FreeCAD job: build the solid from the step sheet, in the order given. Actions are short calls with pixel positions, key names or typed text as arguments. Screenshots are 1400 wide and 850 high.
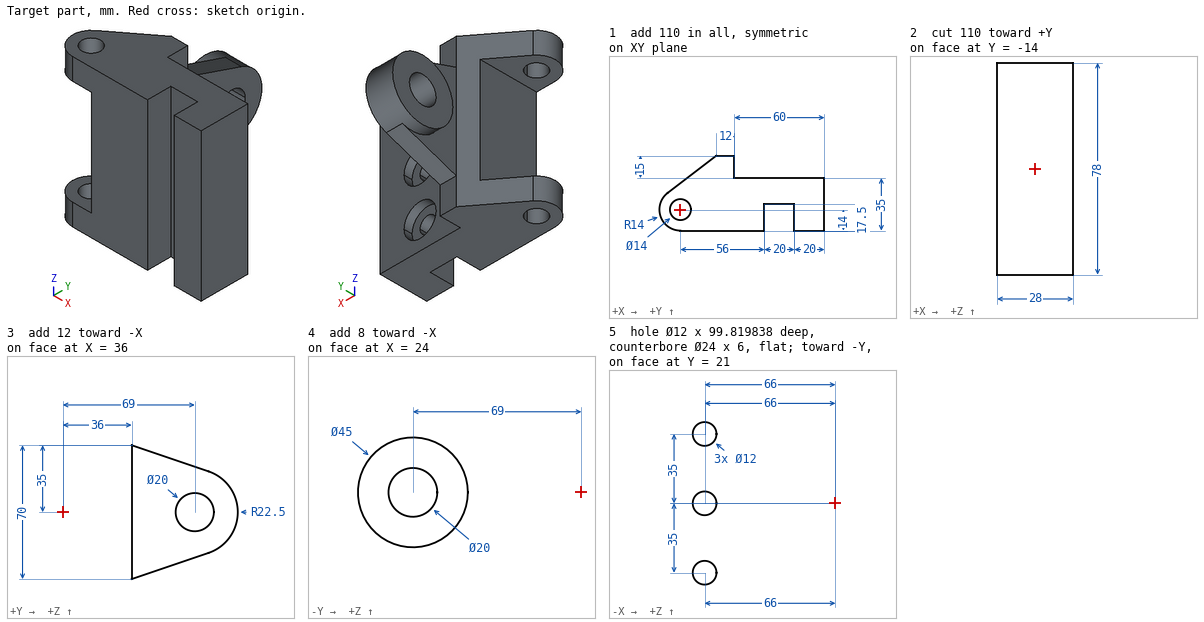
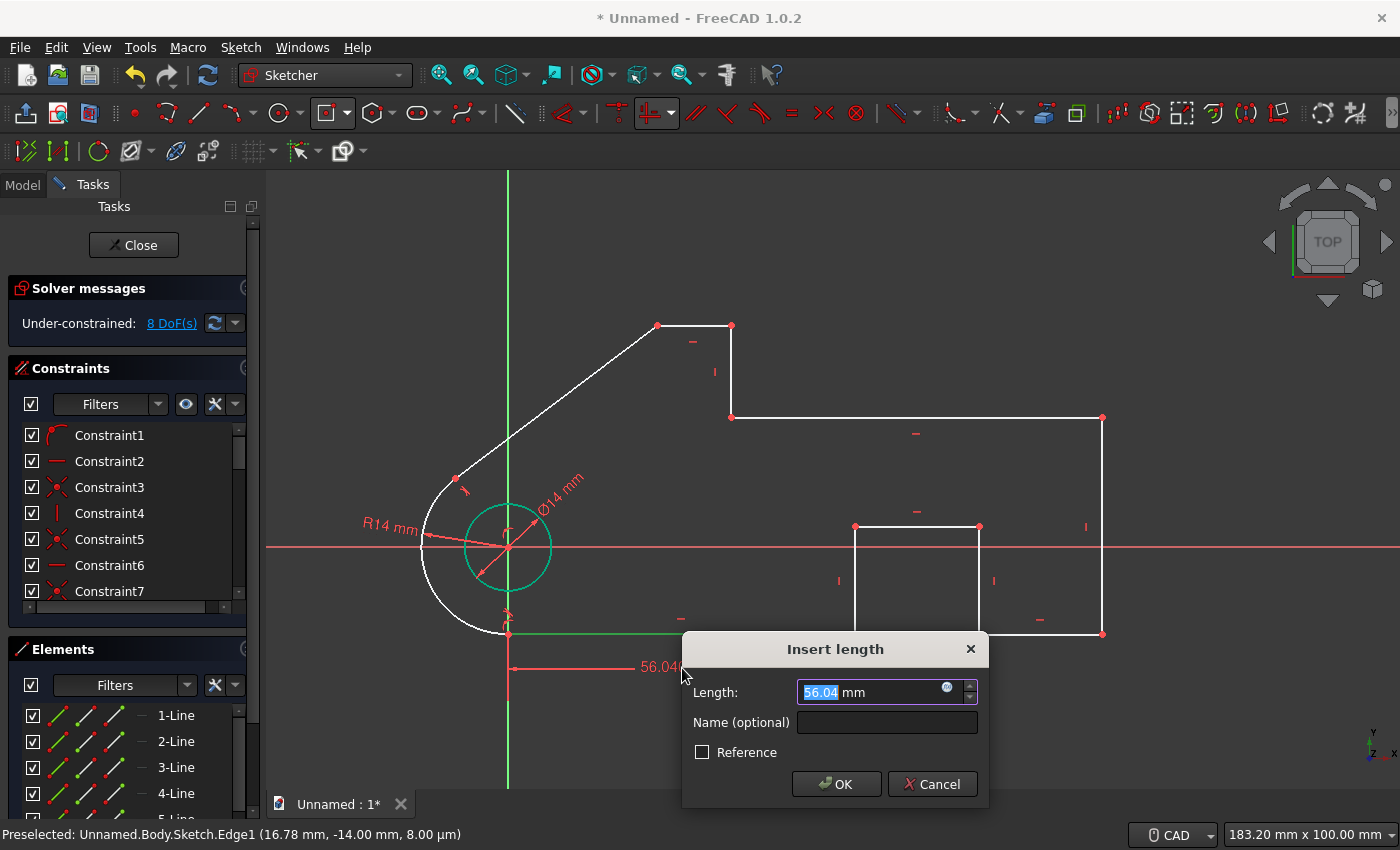
text(56)
key(Return)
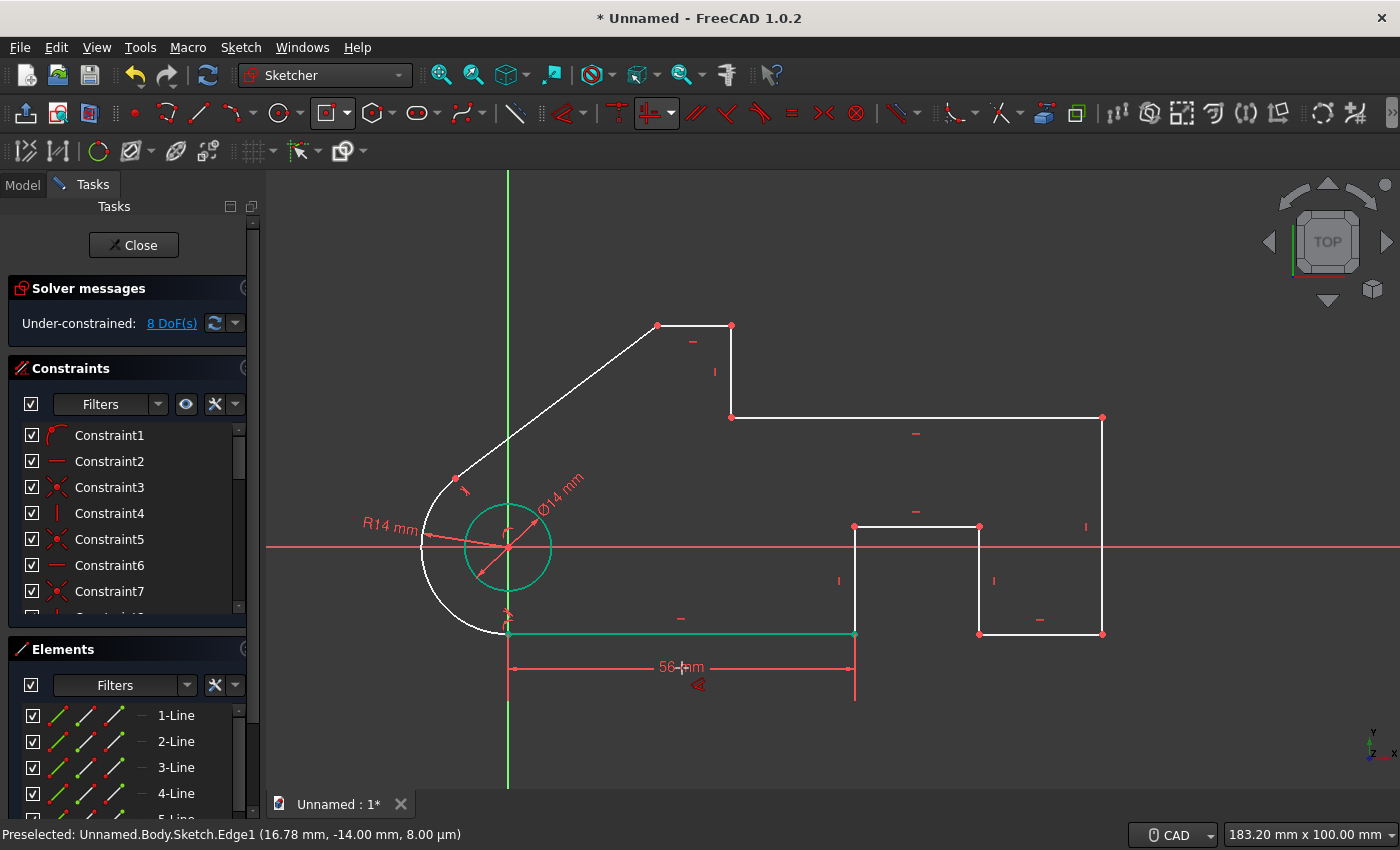
click(892, 527)
click(917, 561)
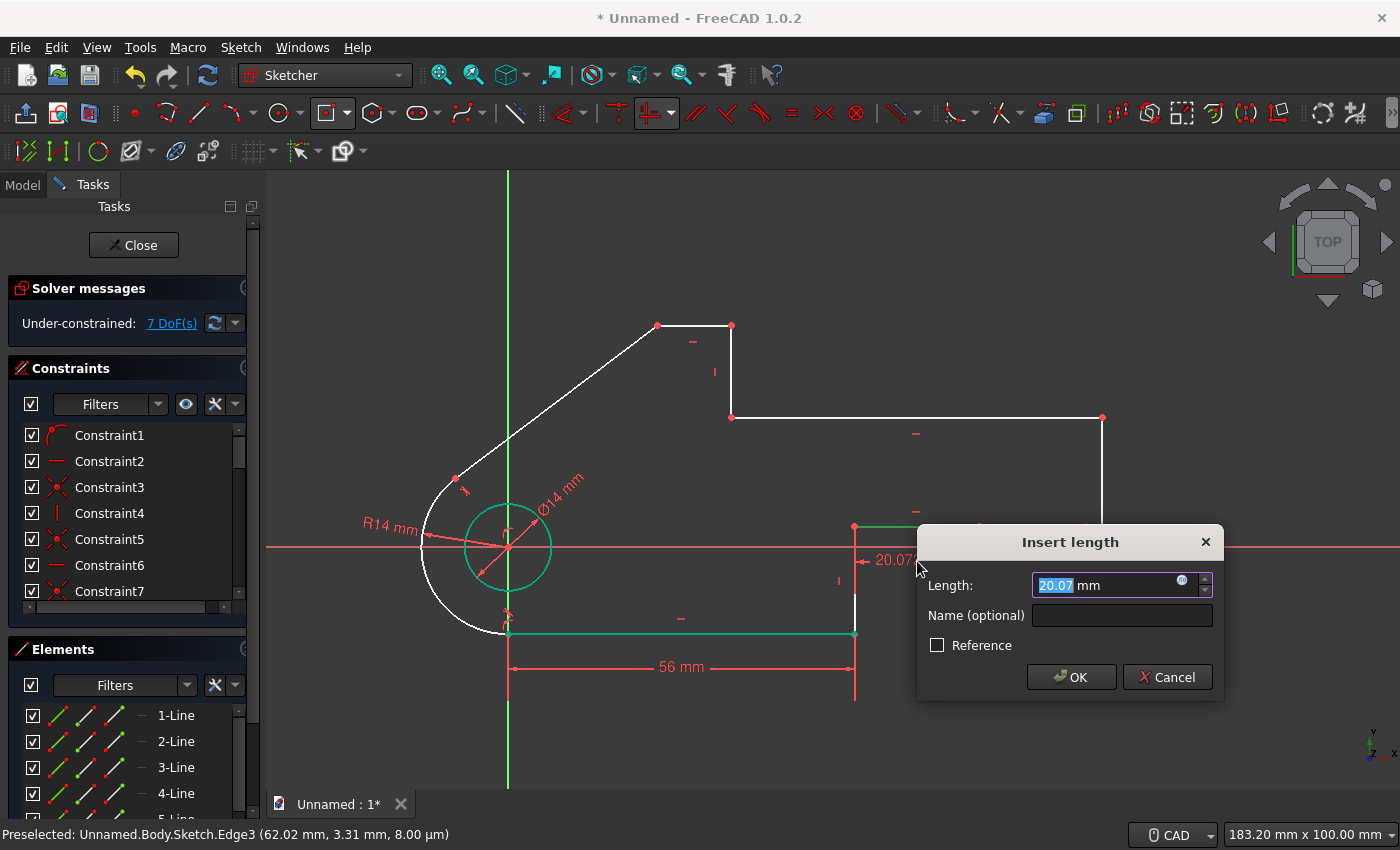
text(20)
key(Return)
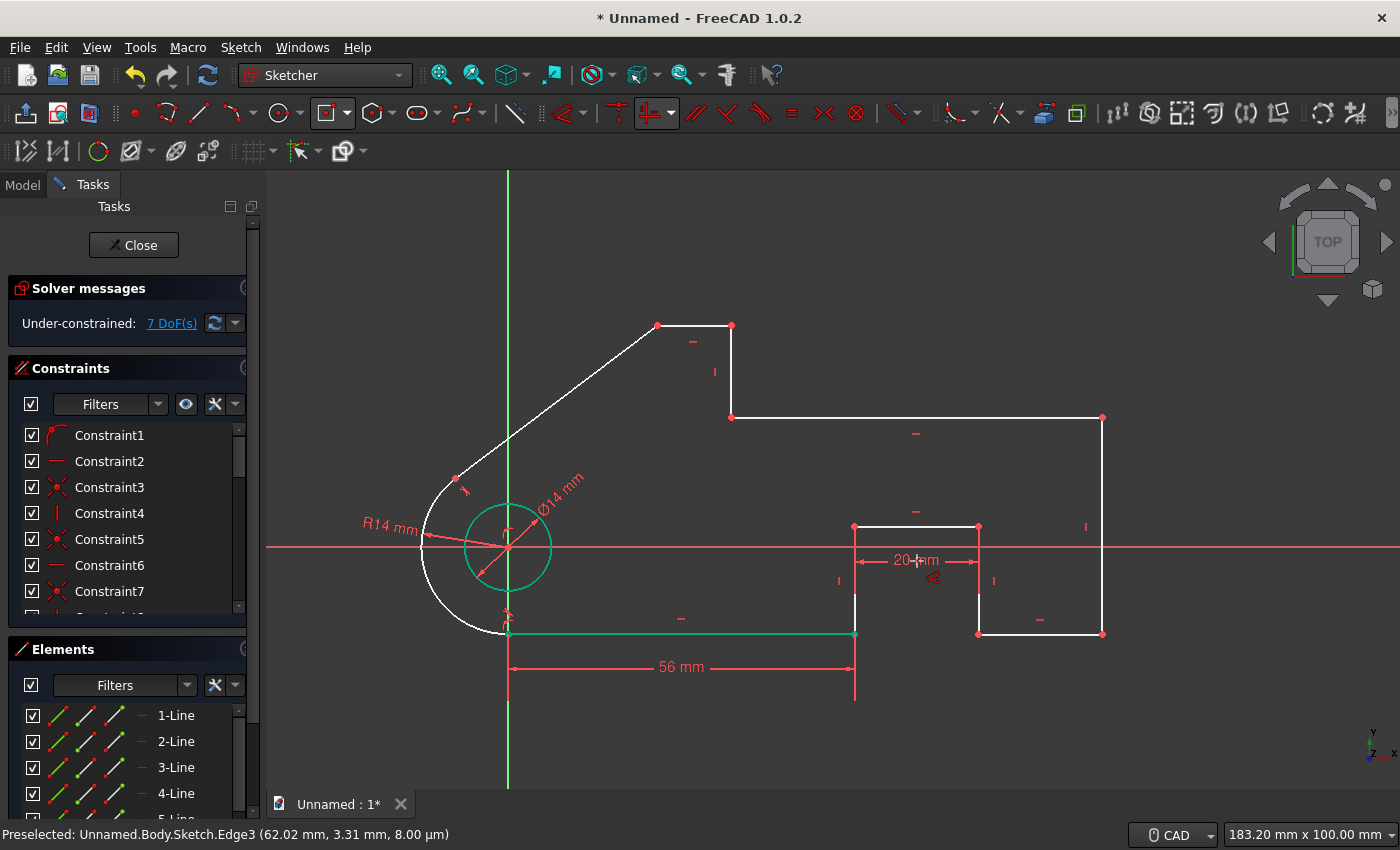
click(1016, 635)
click(1040, 669)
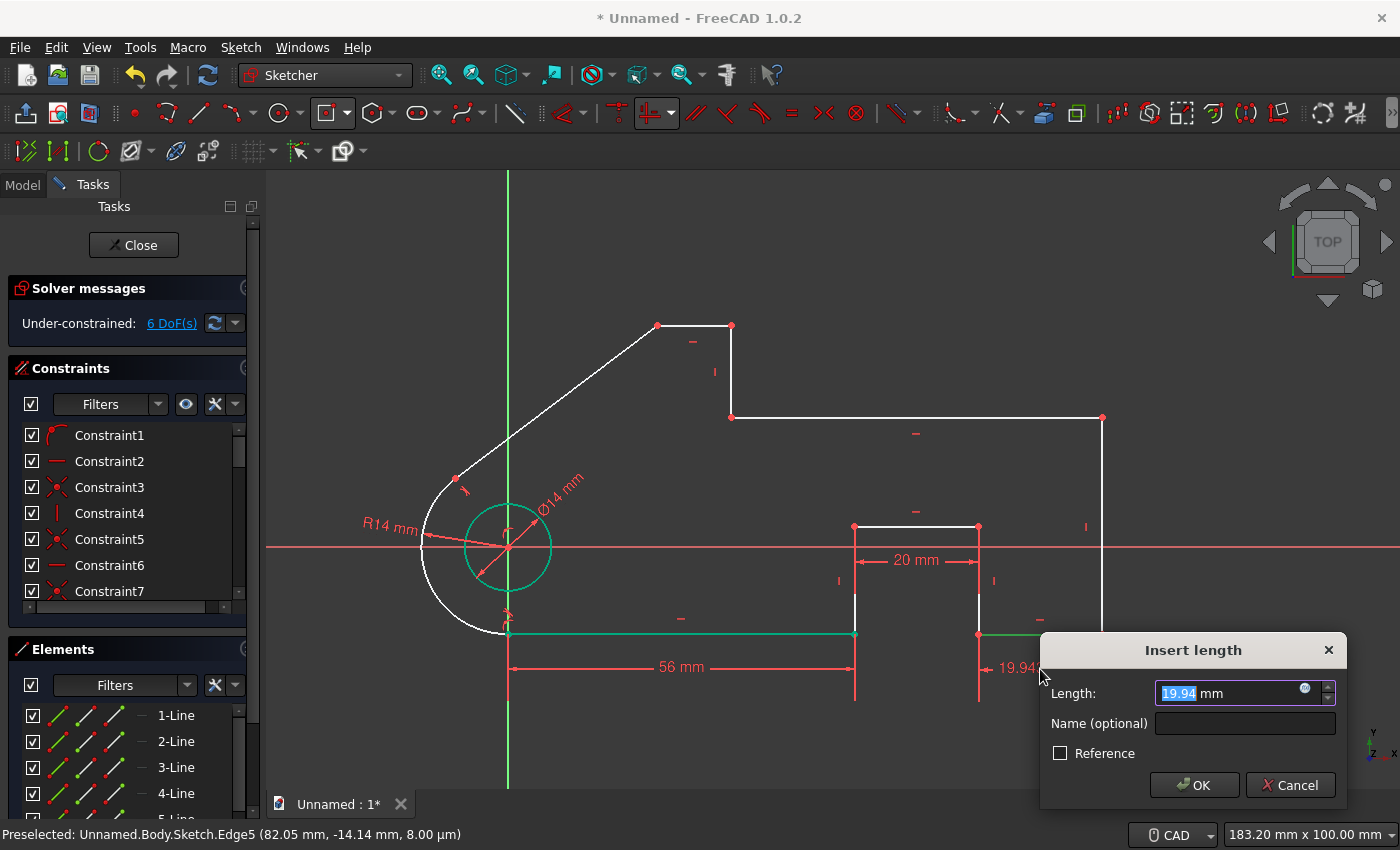
text(20)
key(Return)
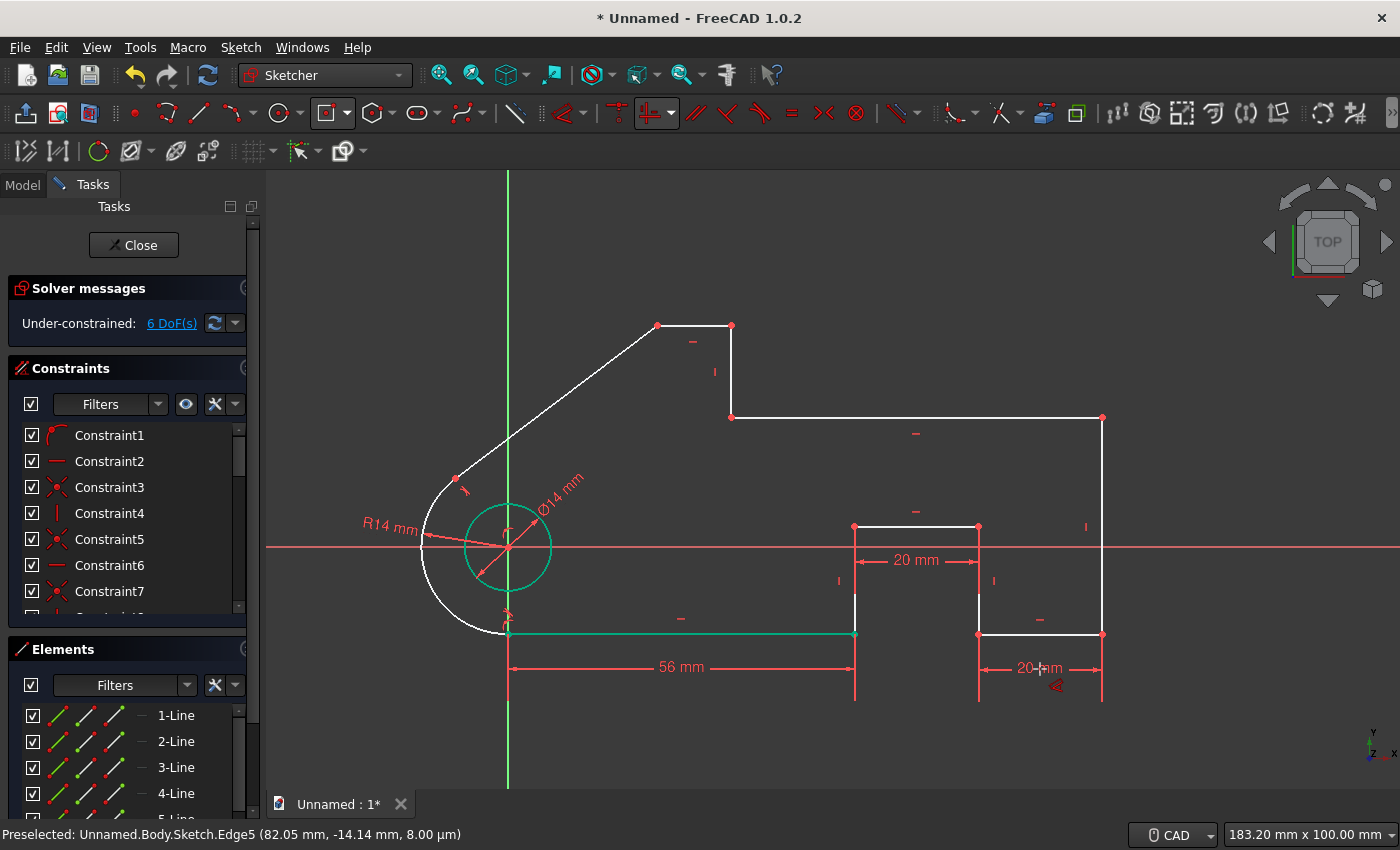
click(1102, 570)
click(1136, 527)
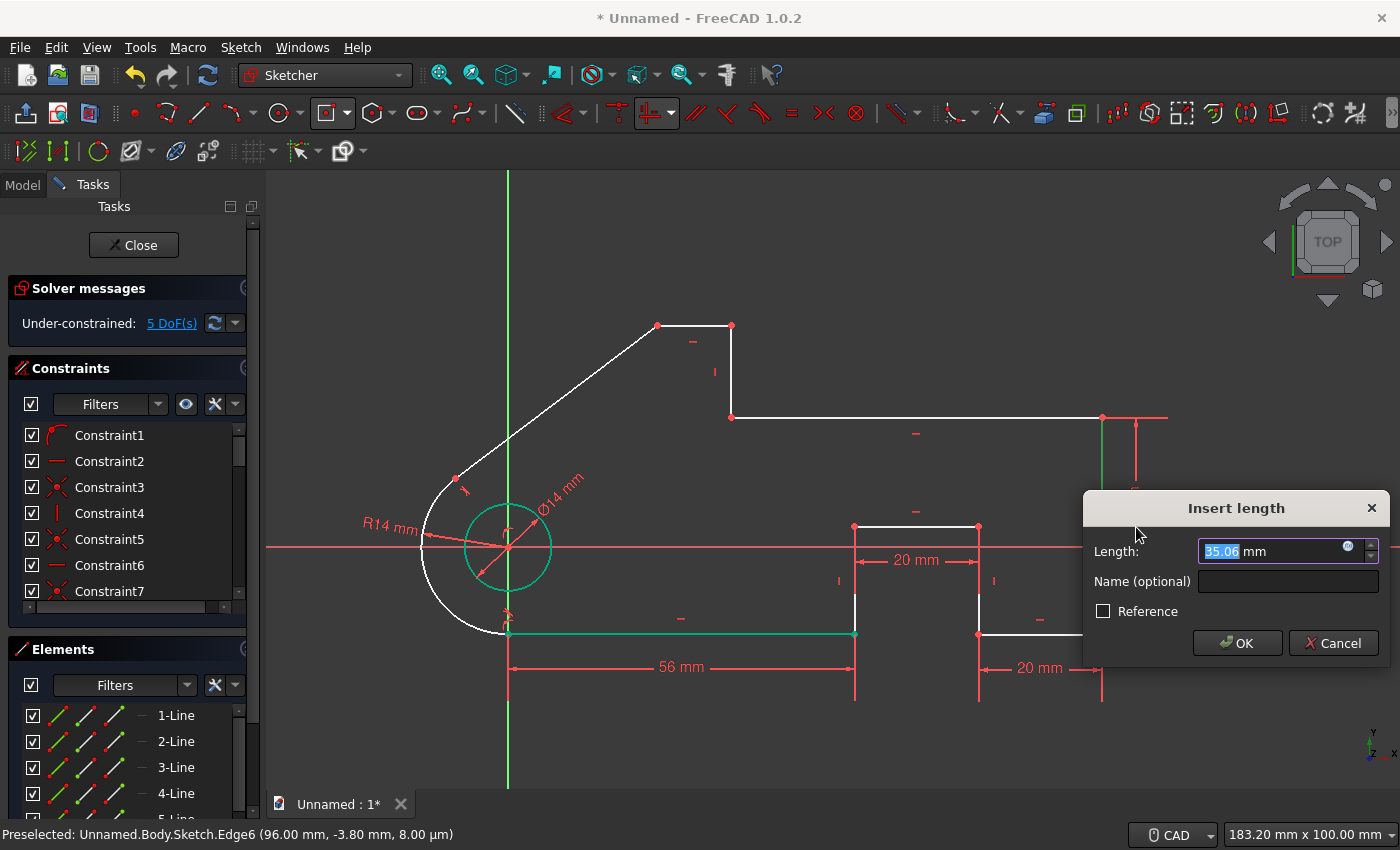
text(35)
key(Return)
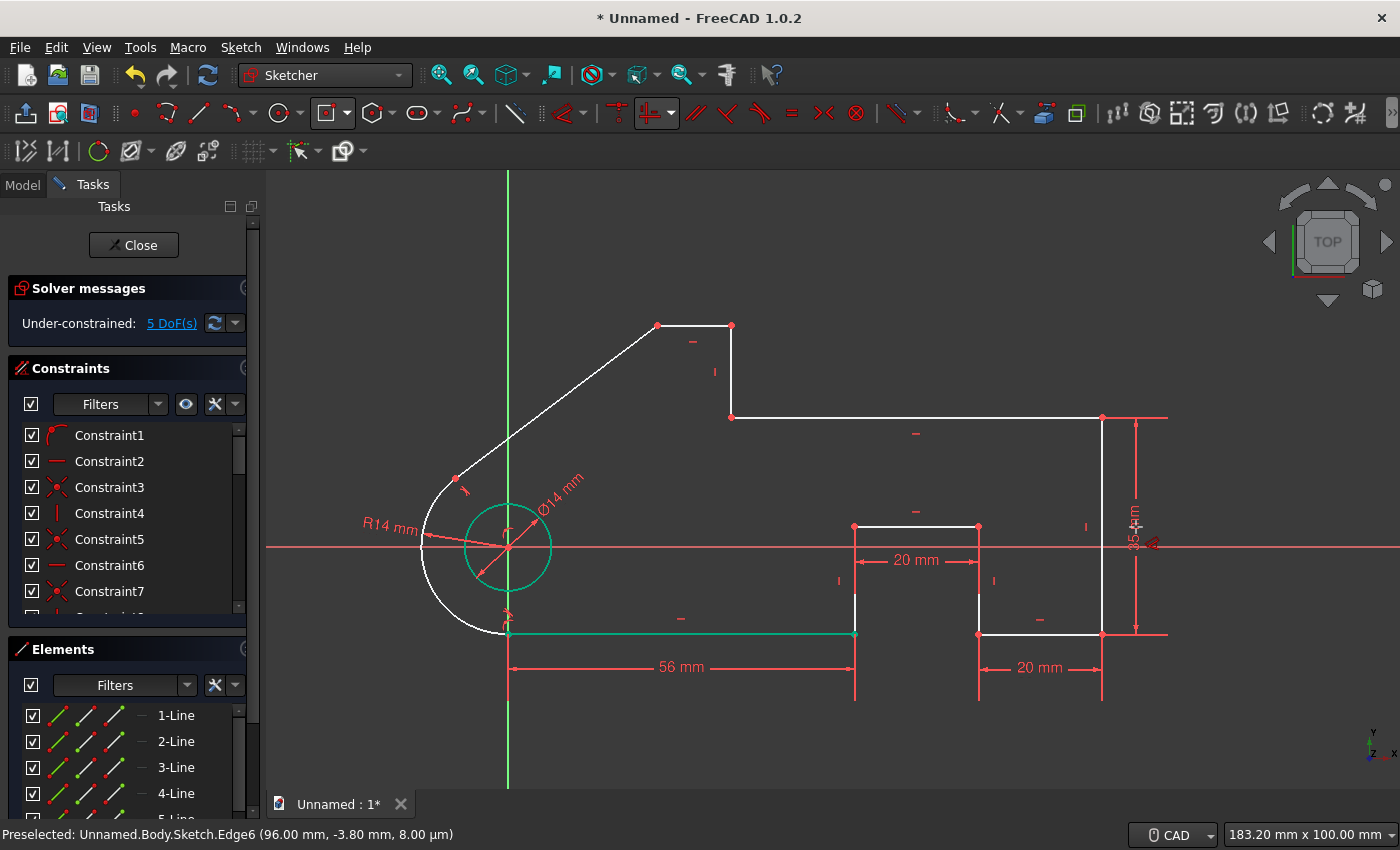
click(991, 418)
click(917, 384)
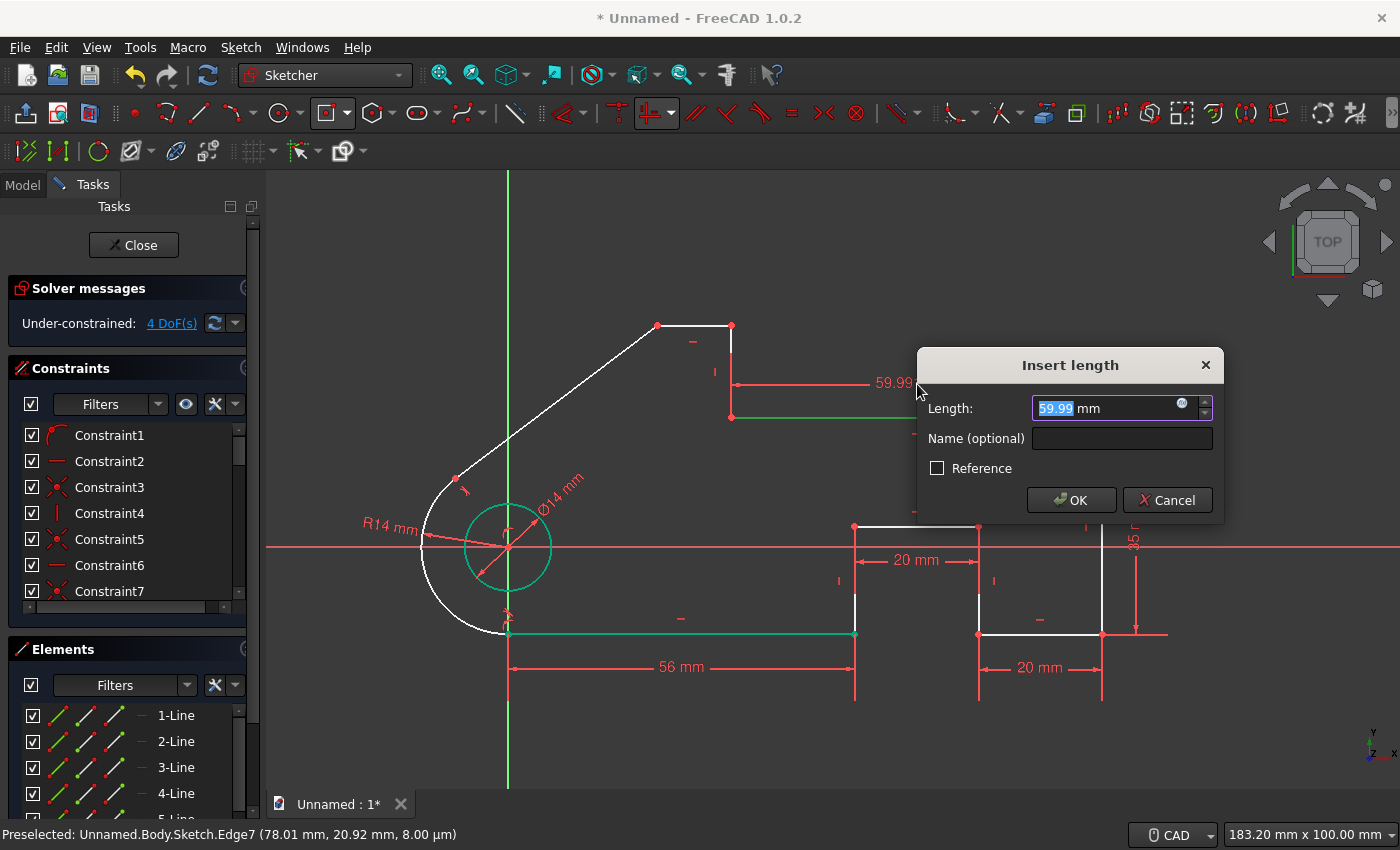
text(60)
key(Return)